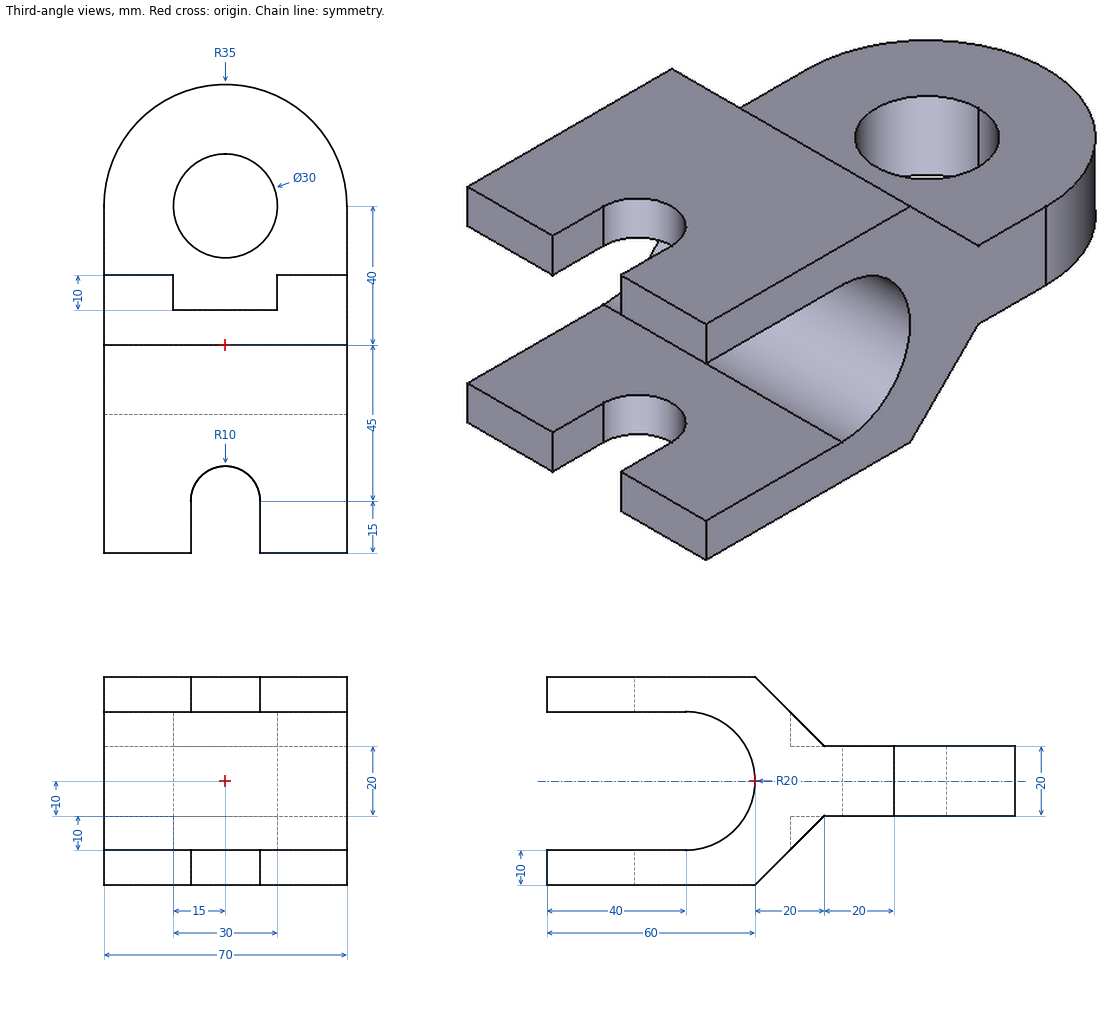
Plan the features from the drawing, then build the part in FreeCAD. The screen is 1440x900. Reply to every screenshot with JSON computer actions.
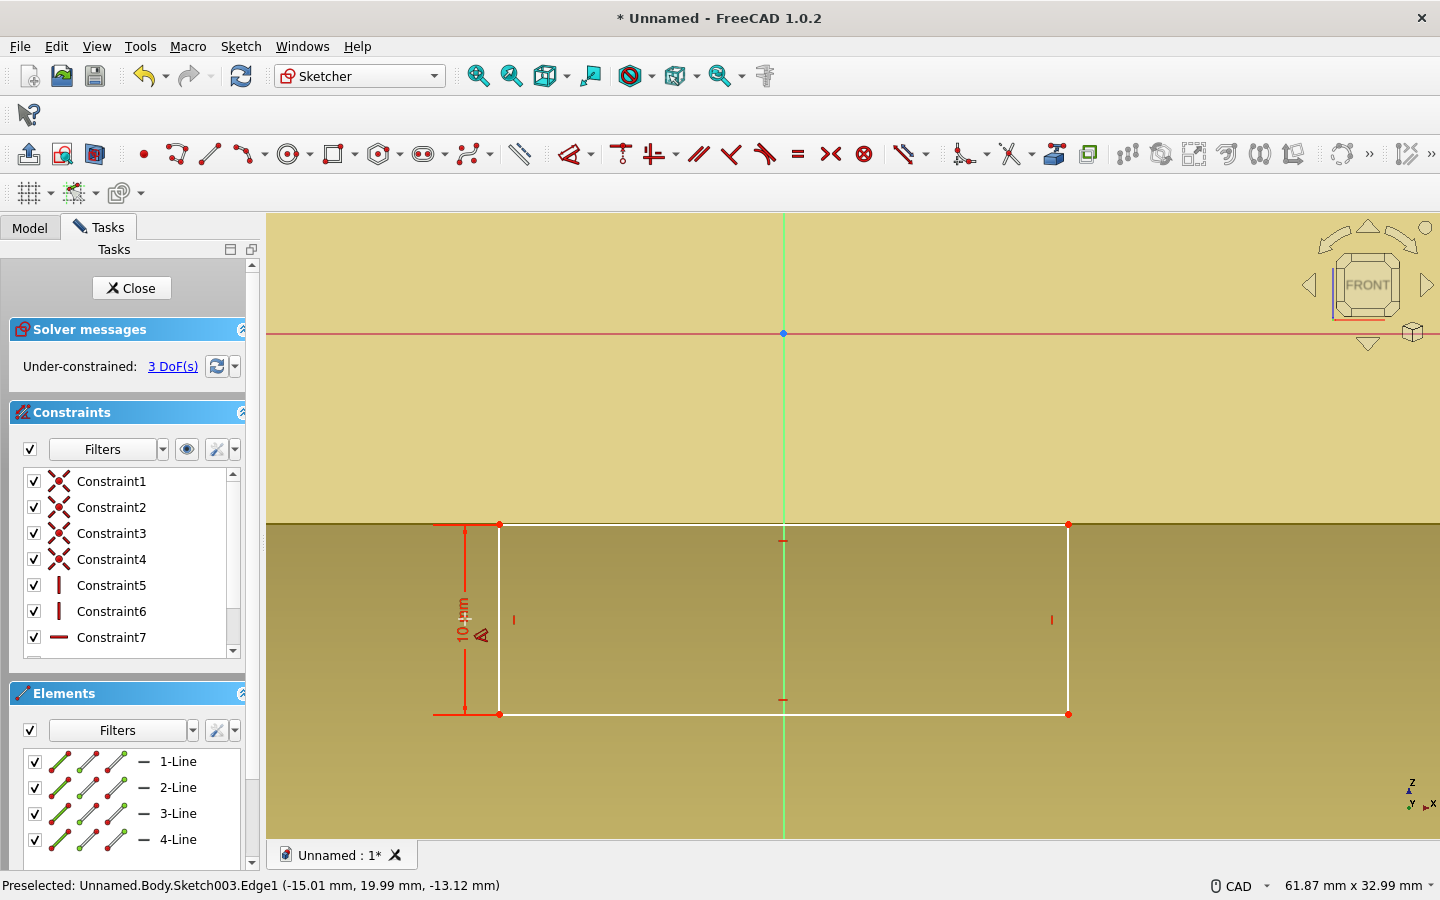
{"action": "left_click", "coordinate": [670, 715]}
{"action": "left_click", "coordinate": [653, 749]}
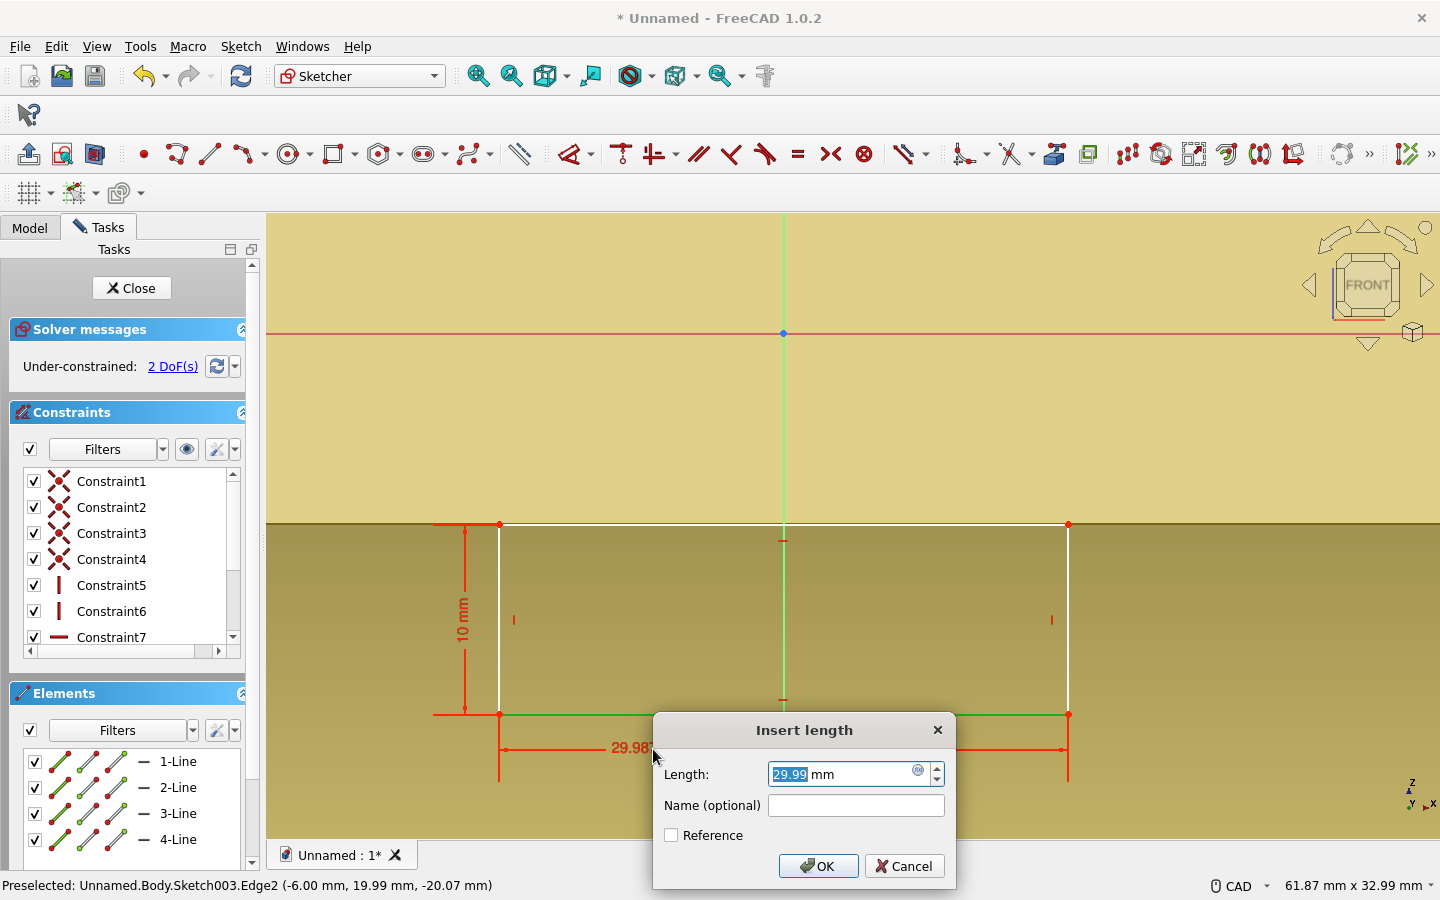
{"action": "type", "text": "30"}
{"action": "key", "text": "Return"}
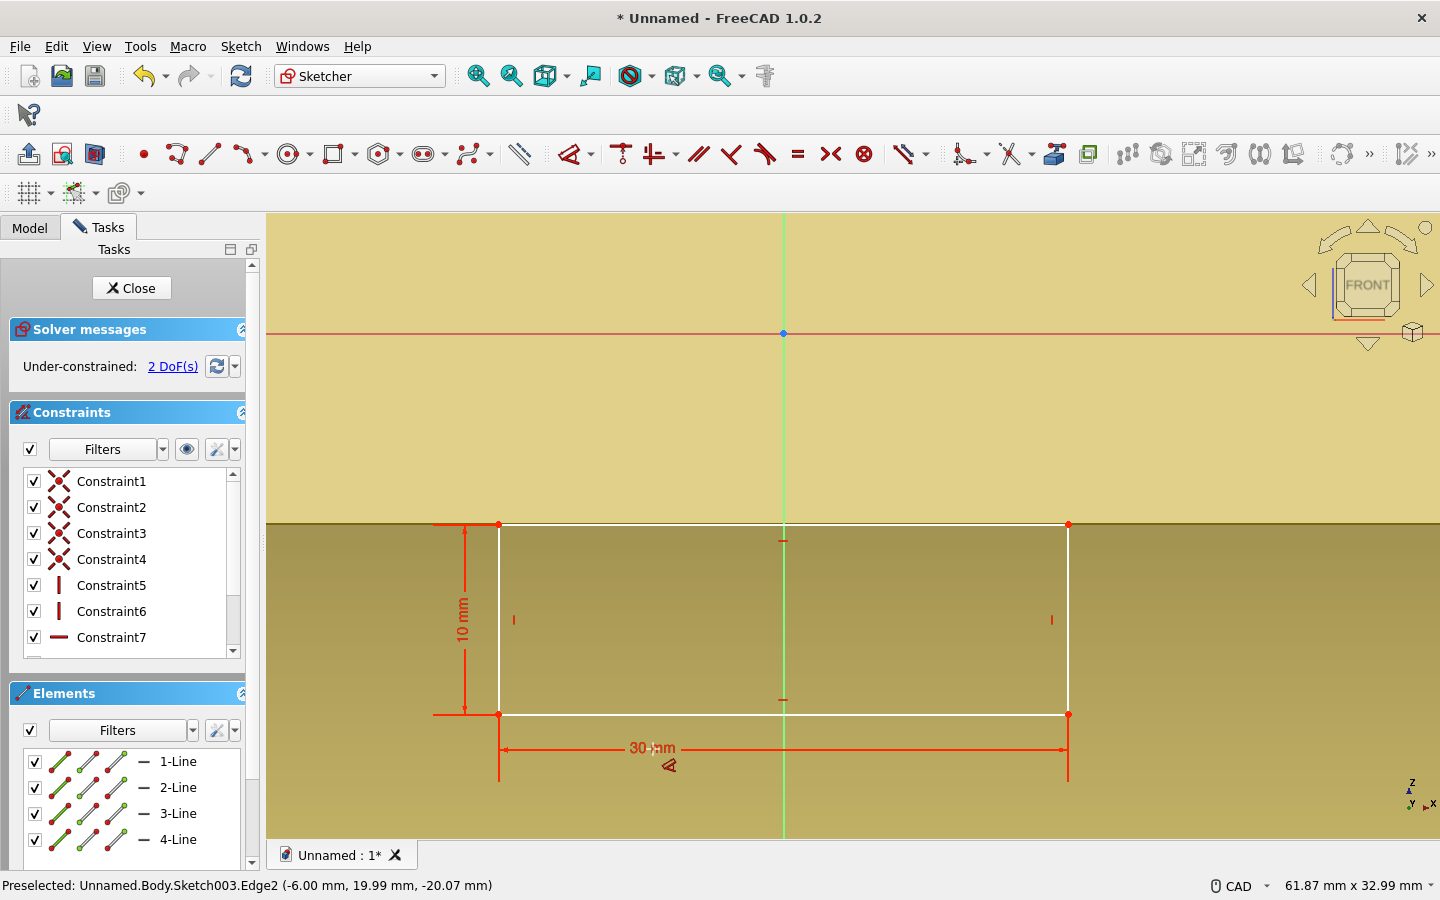
{"action": "left_click", "coordinate": [499, 525]}
{"action": "left_click", "coordinate": [641, 300]}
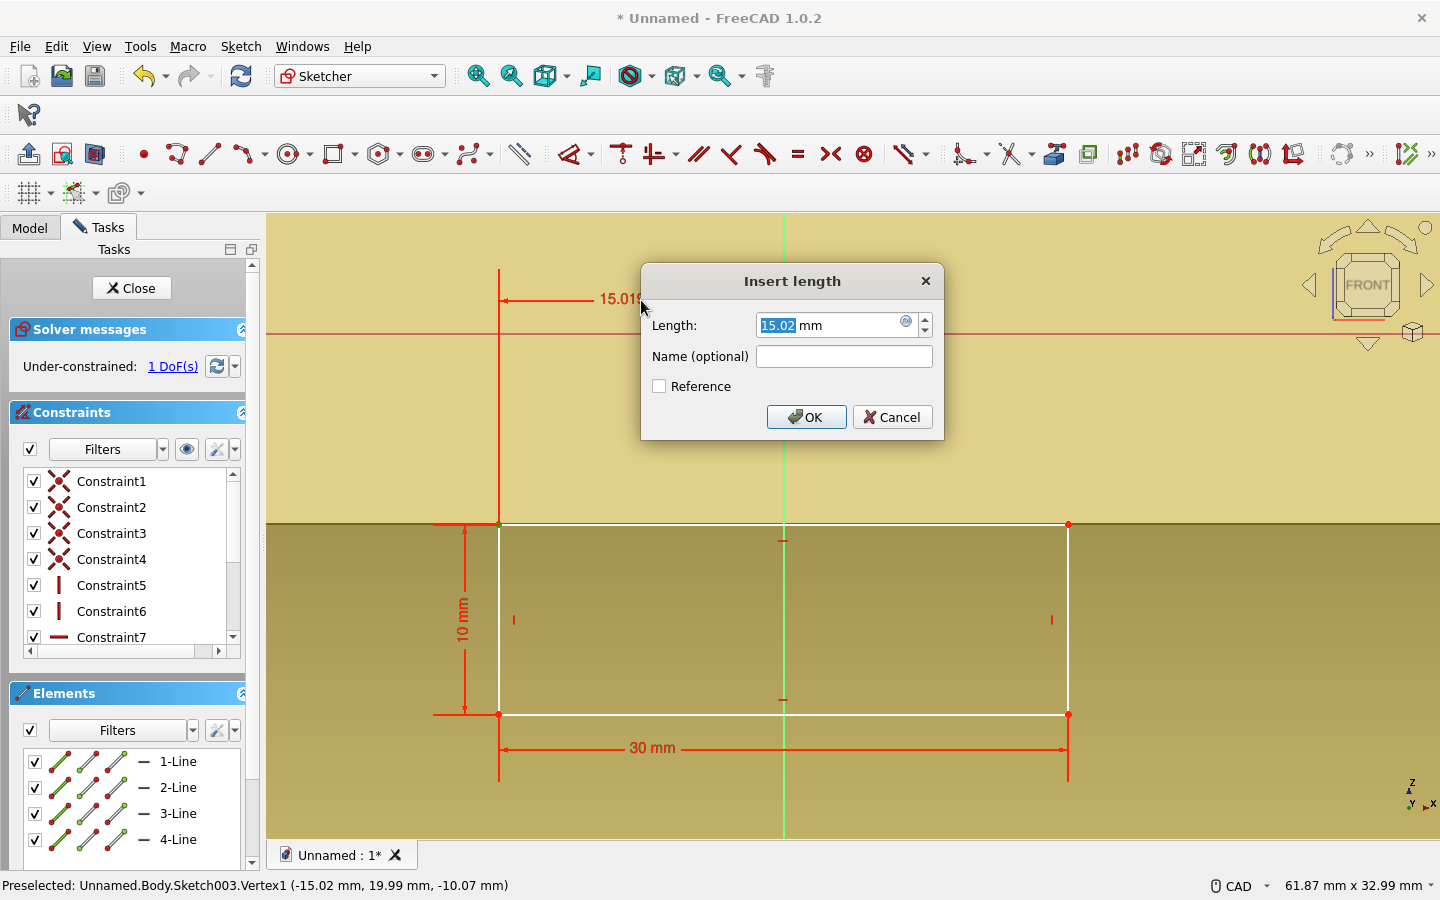
{"action": "type", "text": "15"}
{"action": "key", "text": "Return"}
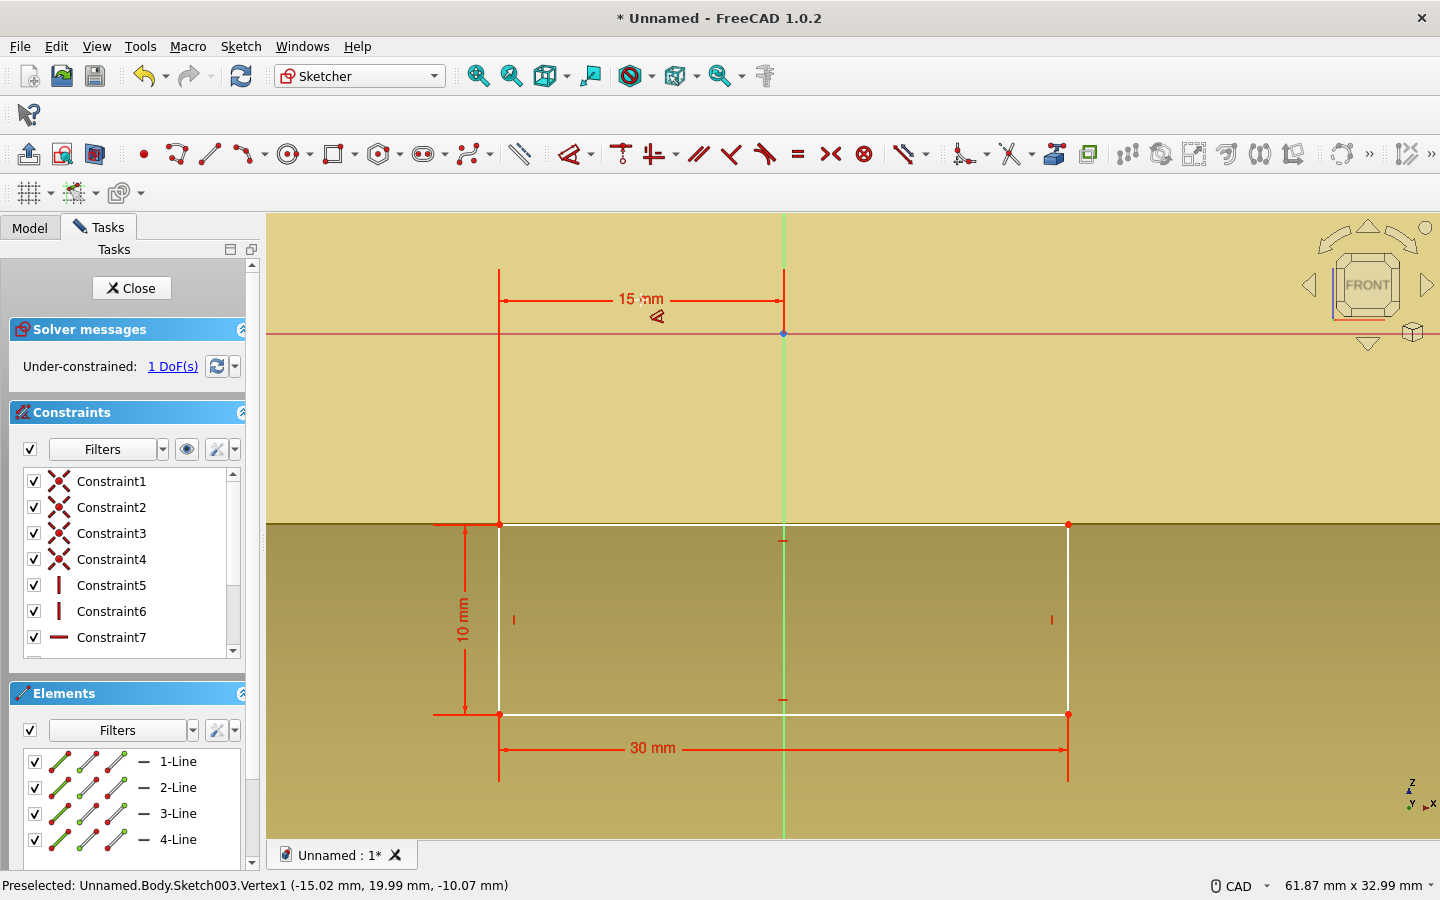
{"action": "left_click", "coordinate": [499, 525]}
{"action": "left_click", "coordinate": [465, 429]}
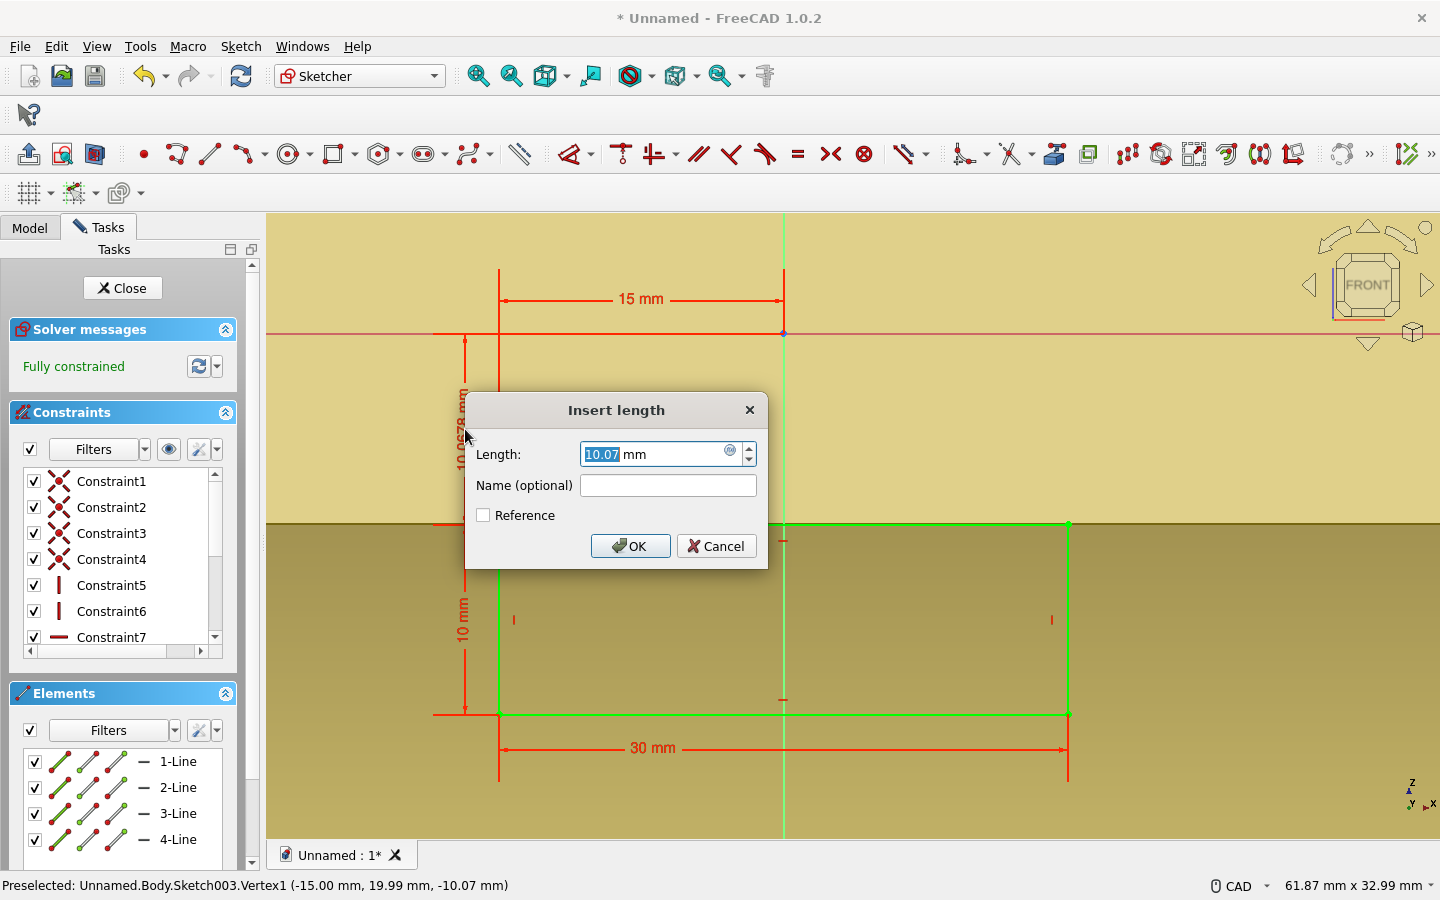
{"action": "type", "text": "10"}
{"action": "key", "text": "Return"}
{"action": "key", "text": "Escape"}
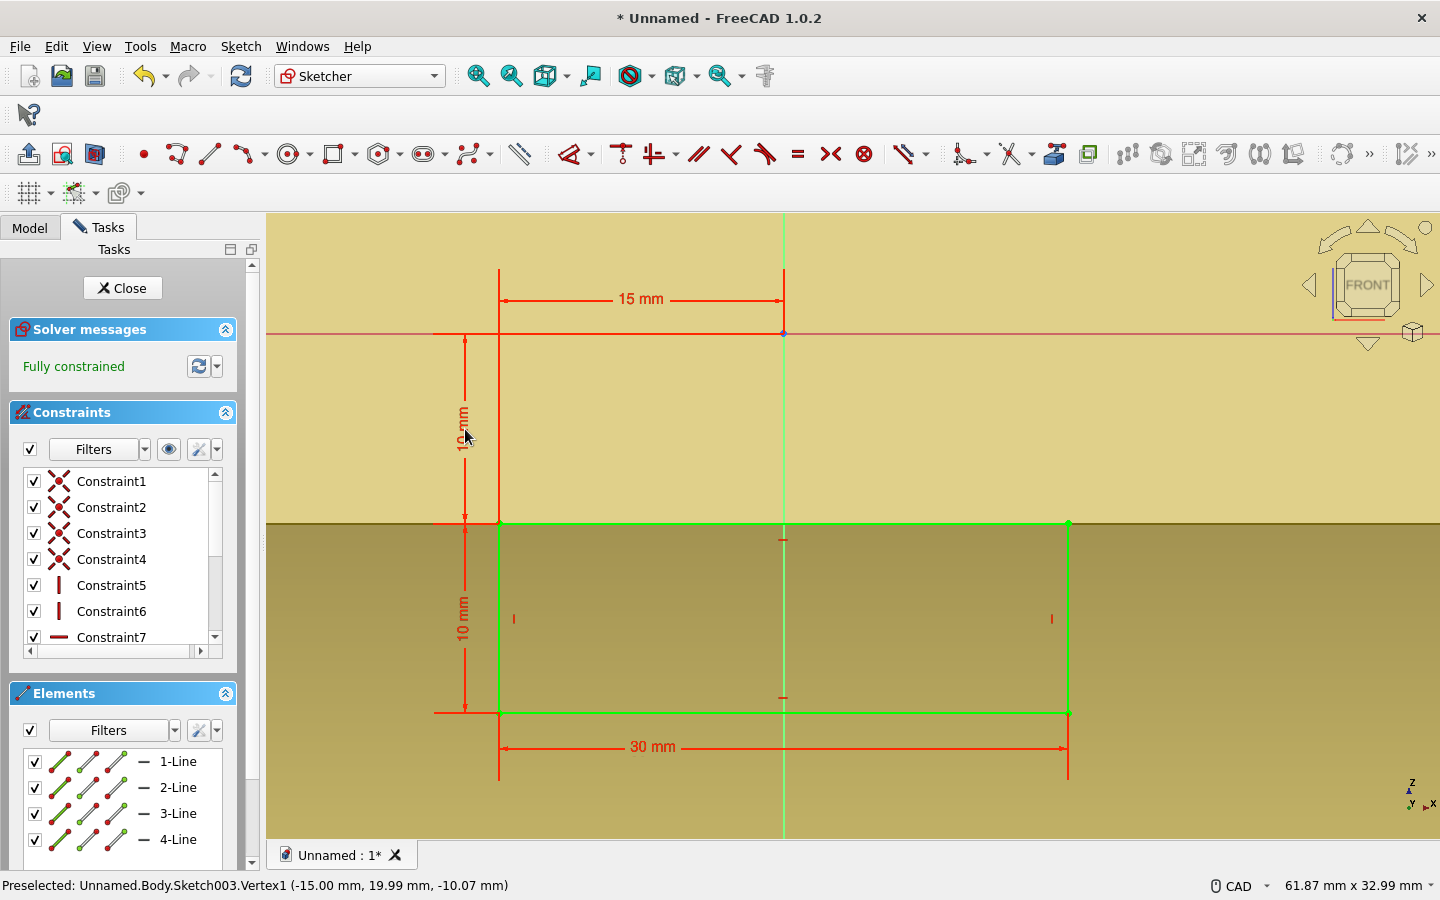
{"action": "left_click", "coordinate": [123, 288]}